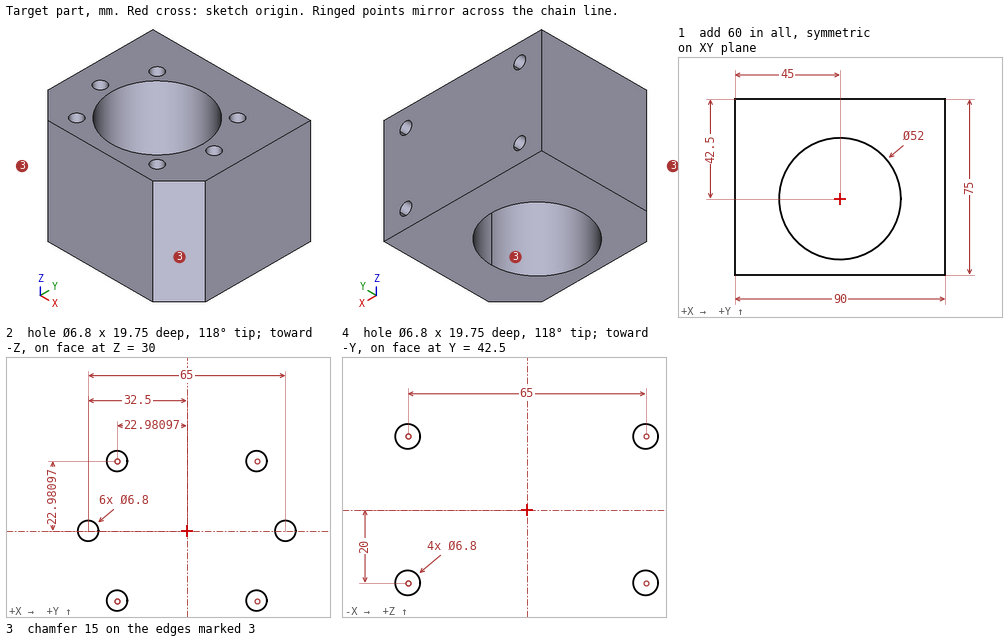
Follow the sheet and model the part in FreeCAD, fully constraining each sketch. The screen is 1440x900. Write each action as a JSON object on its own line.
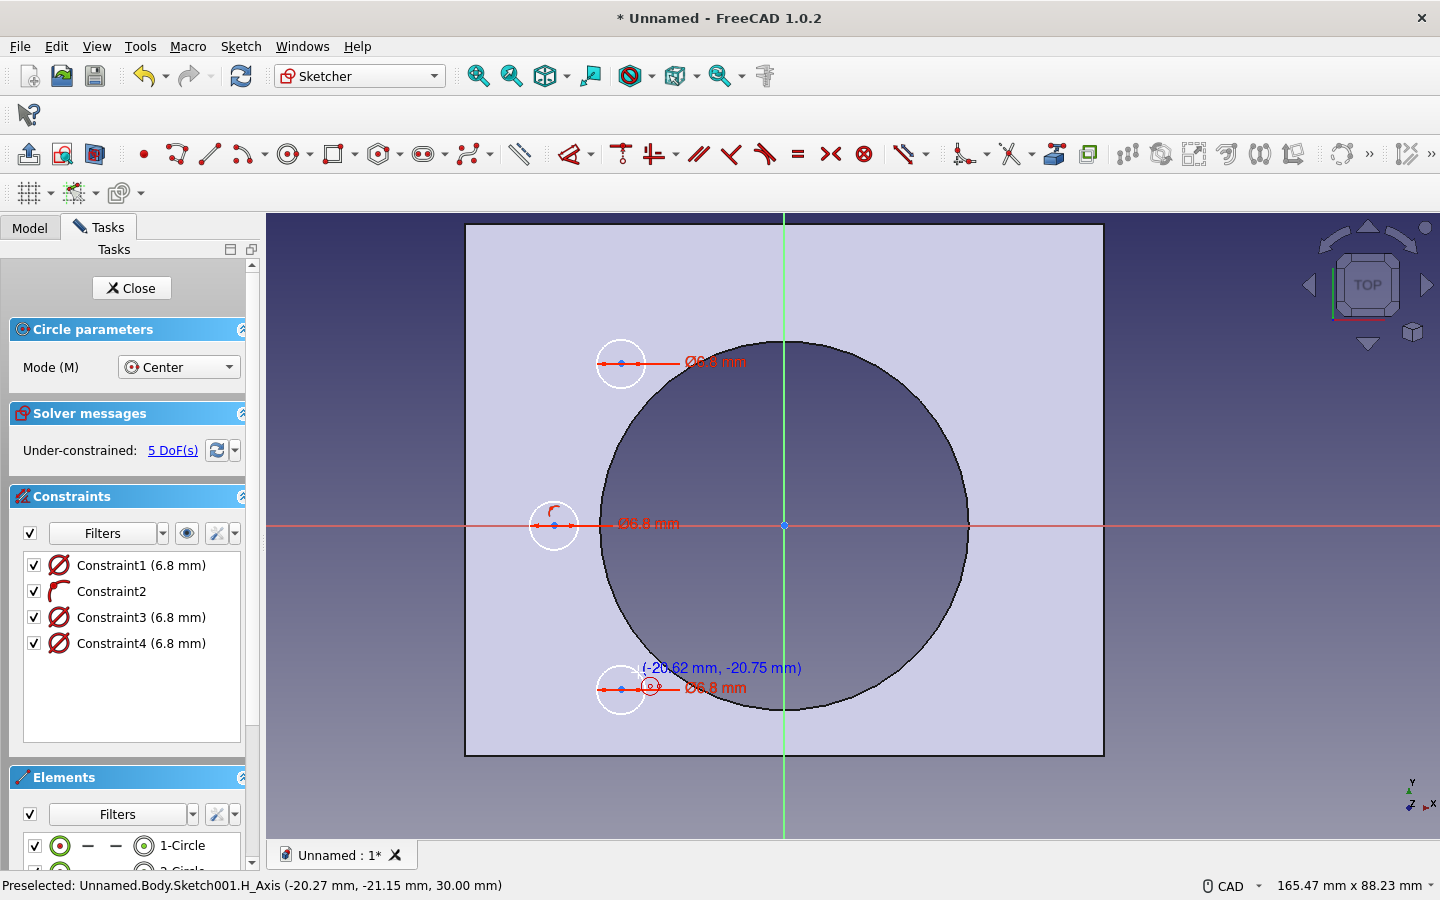
{"action": "left_click", "coordinate": [947, 689]}
{"action": "mouse_move", "coordinate": [964, 672]}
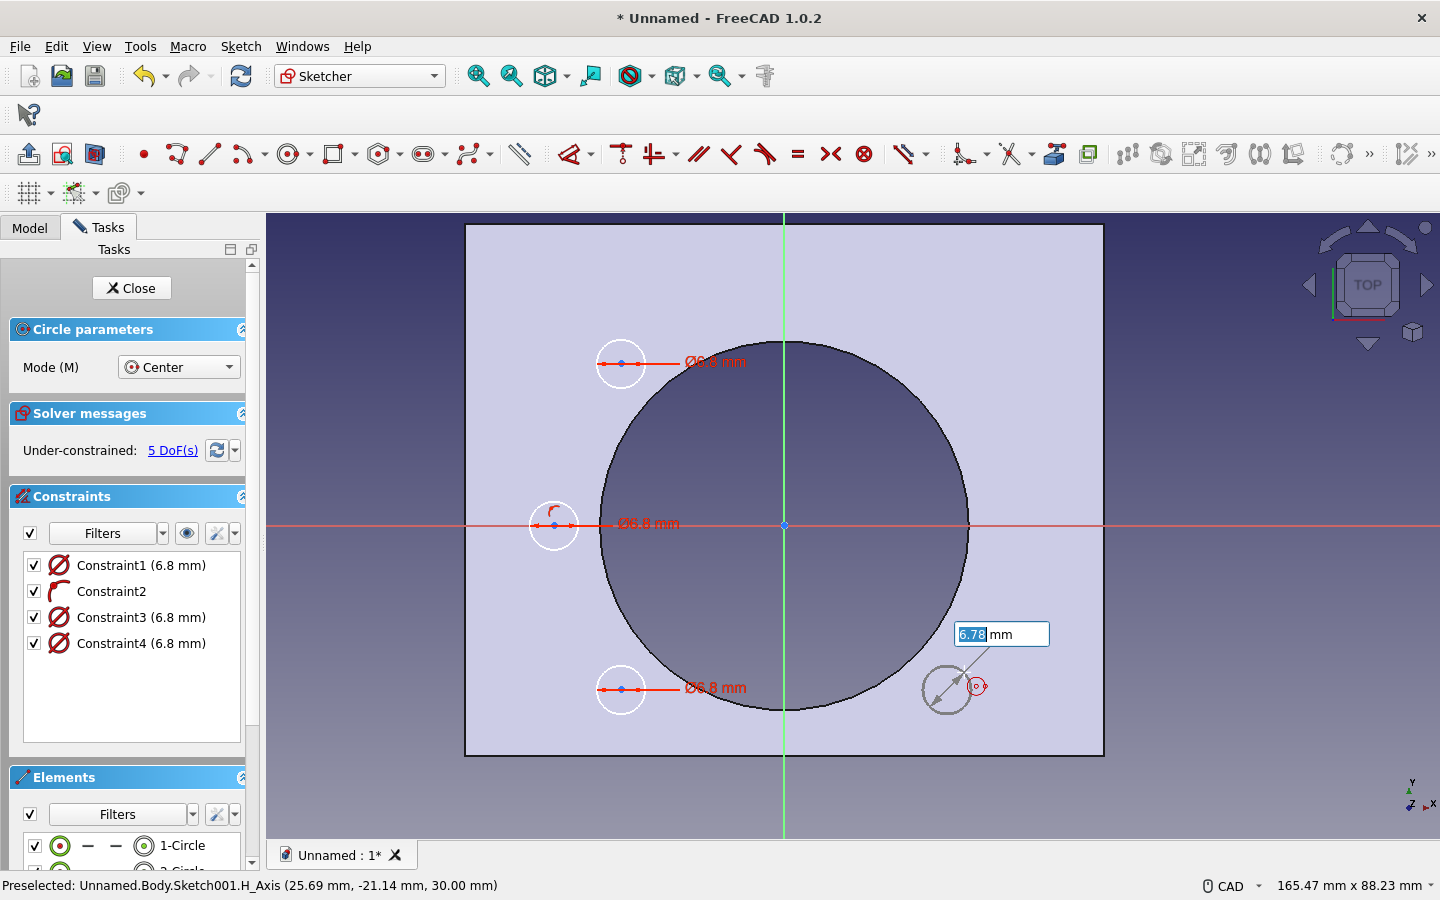
{"action": "type", "text": "6.8"}
{"action": "key", "text": "Return"}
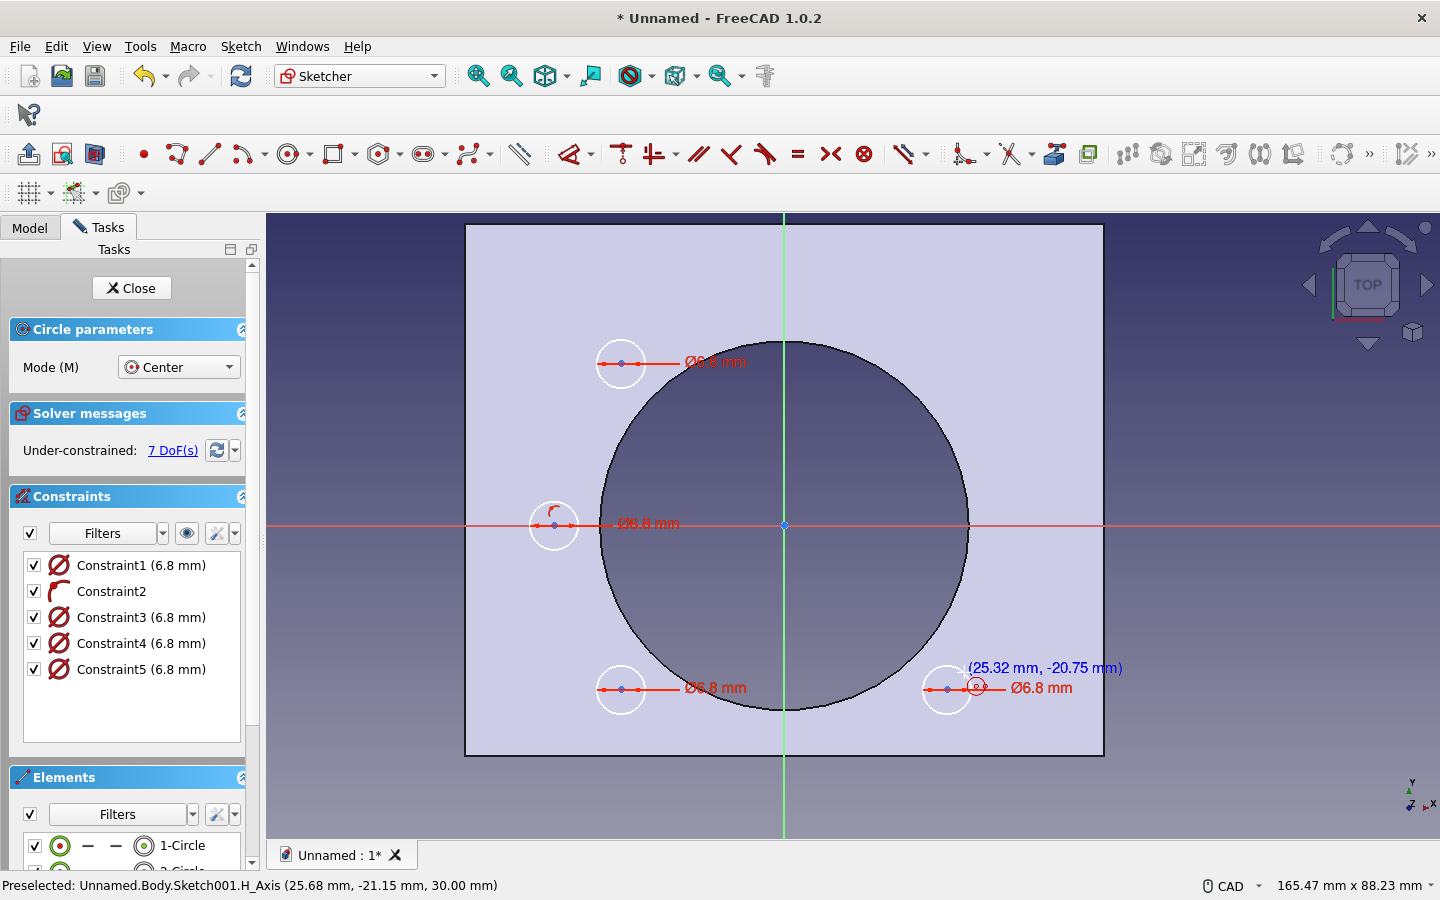
{"action": "left_click", "coordinate": [1015, 526]}
{"action": "mouse_move", "coordinate": [1032, 509]}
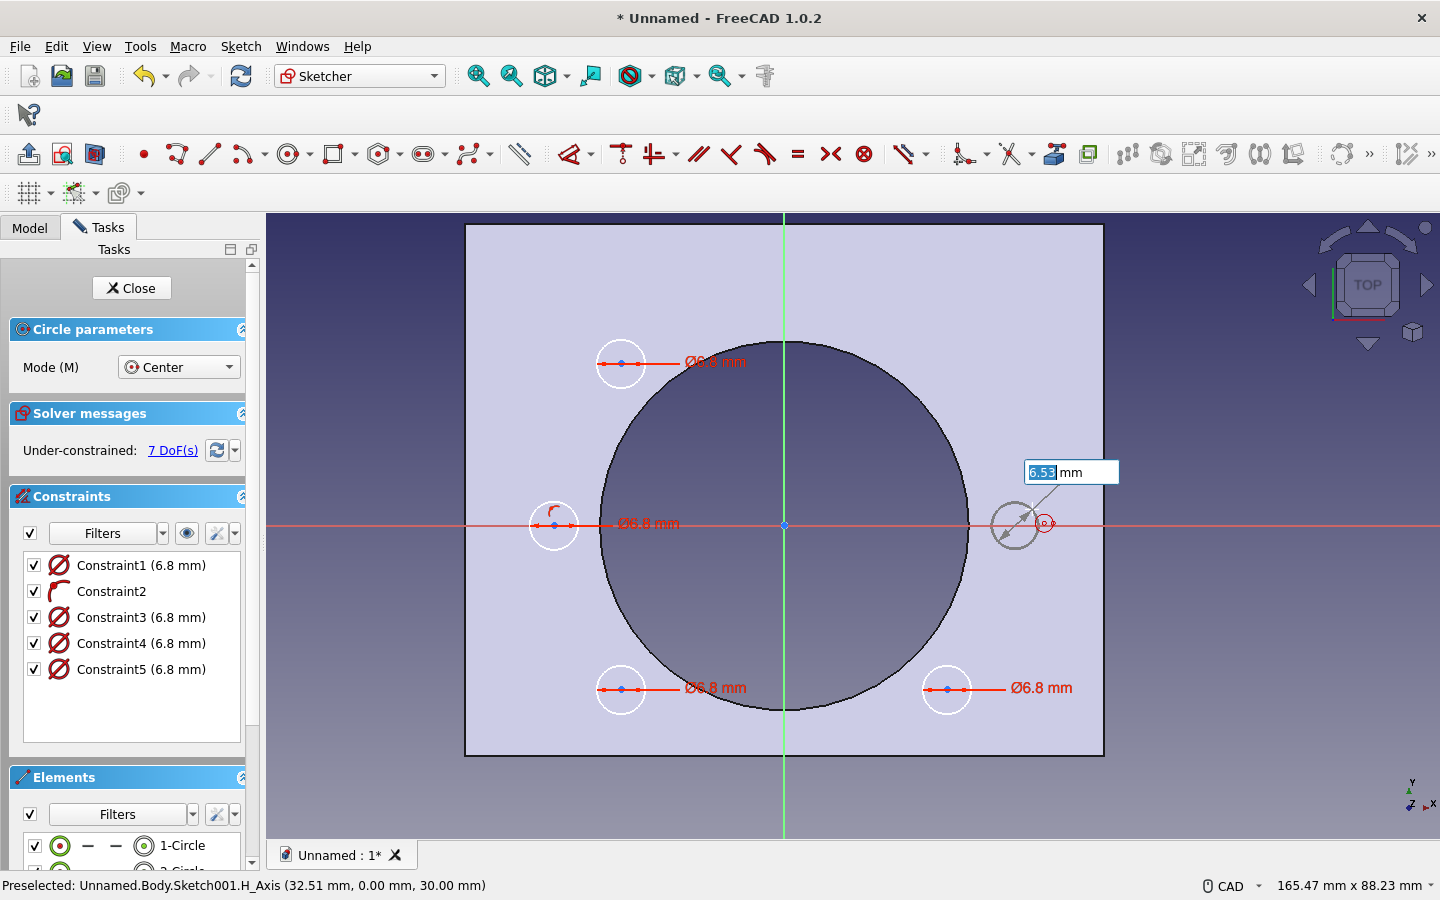
{"action": "type", "text": "6.8"}
{"action": "key", "text": "Return"}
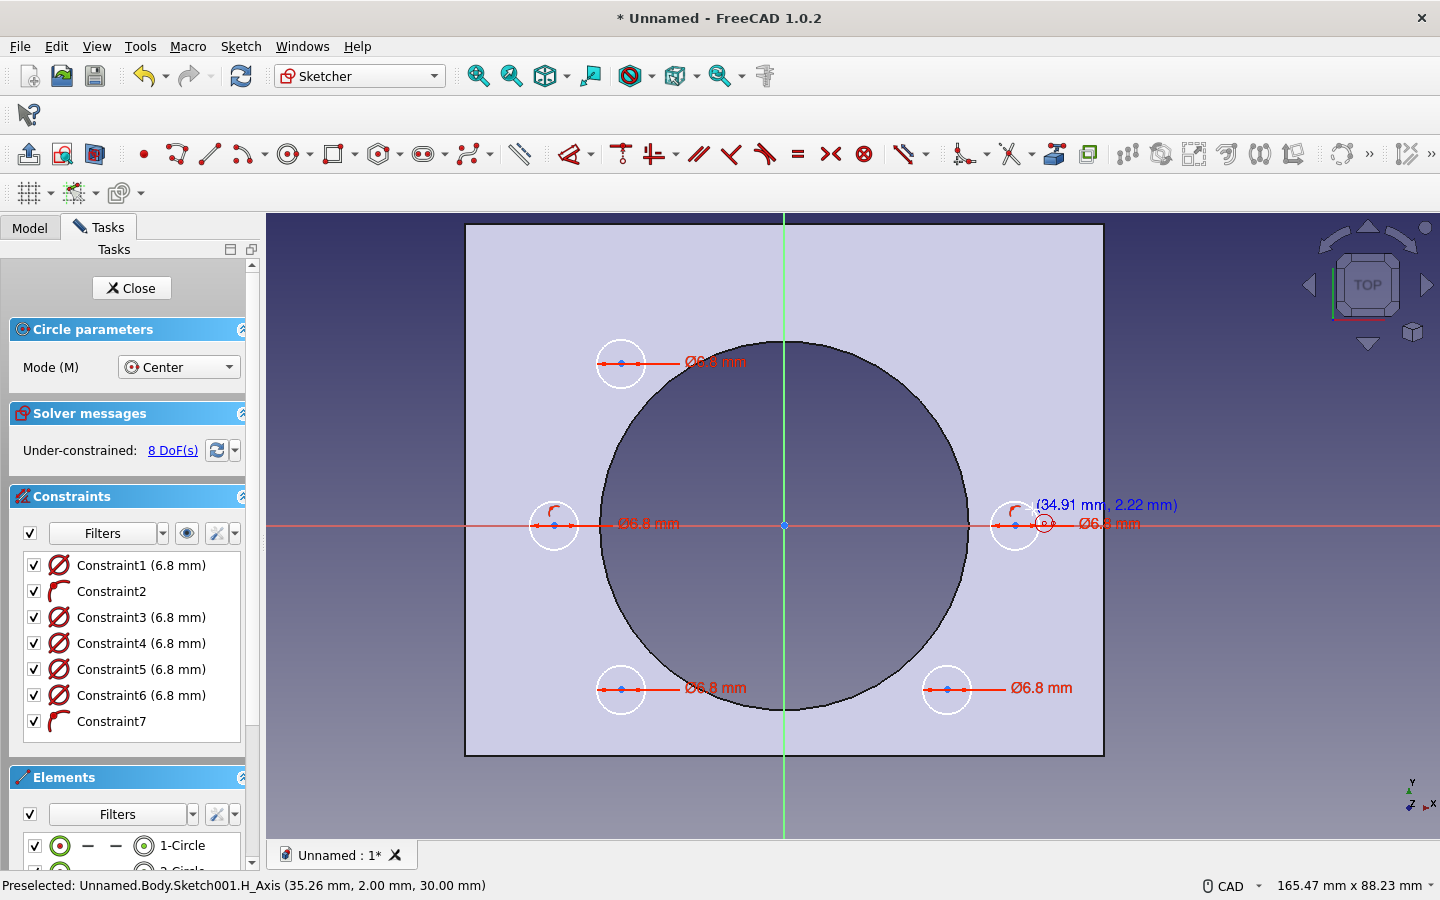
{"action": "left_click", "coordinate": [947, 363]}
{"action": "mouse_move", "coordinate": [964, 346]}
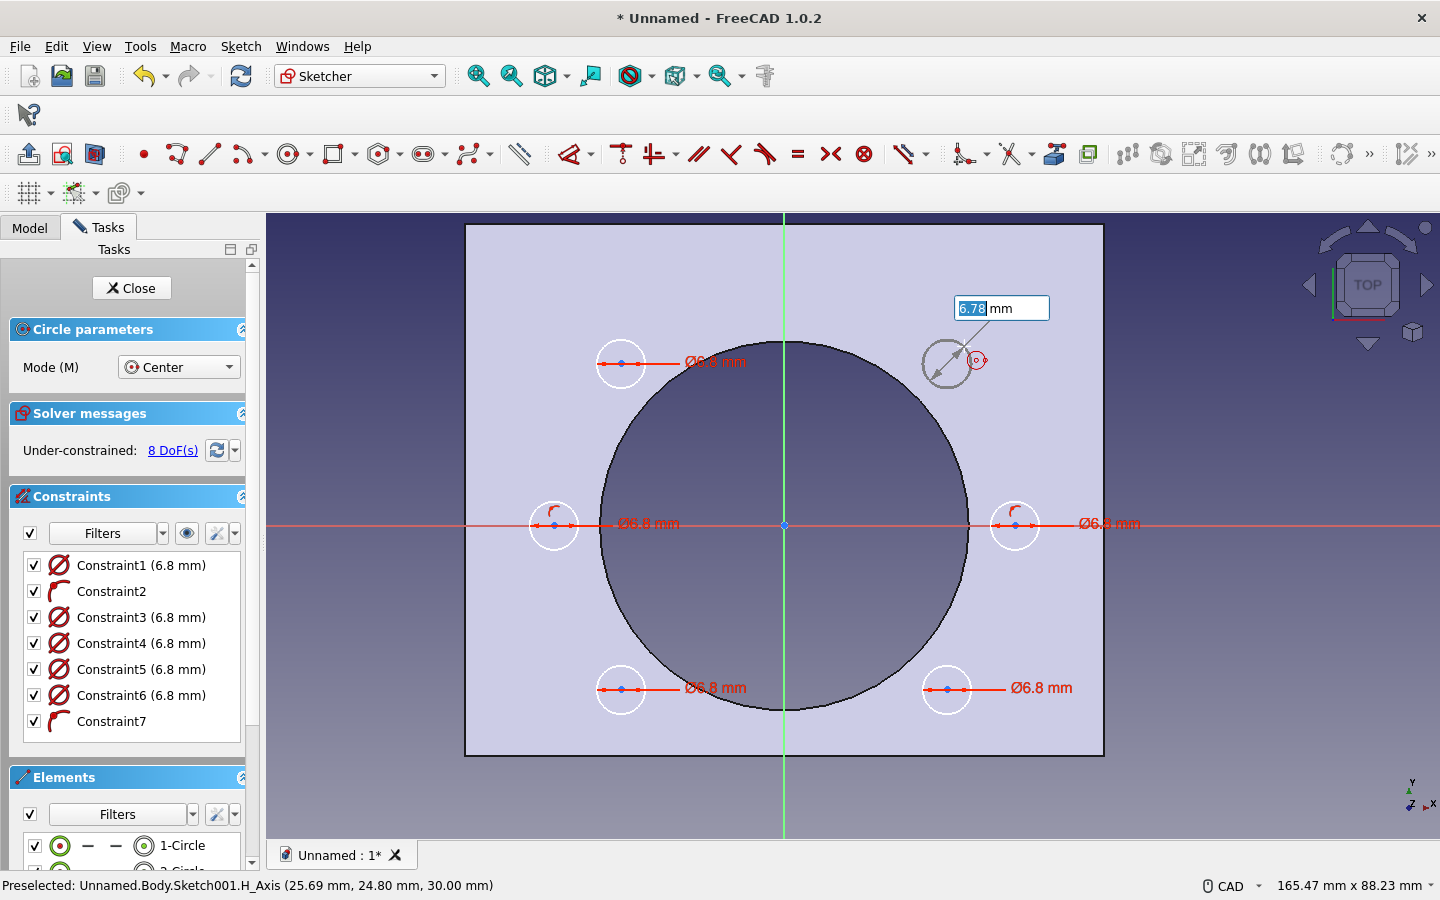
{"action": "type", "text": "6.8"}
{"action": "key", "text": "Return"}
{"action": "key", "text": "Escape"}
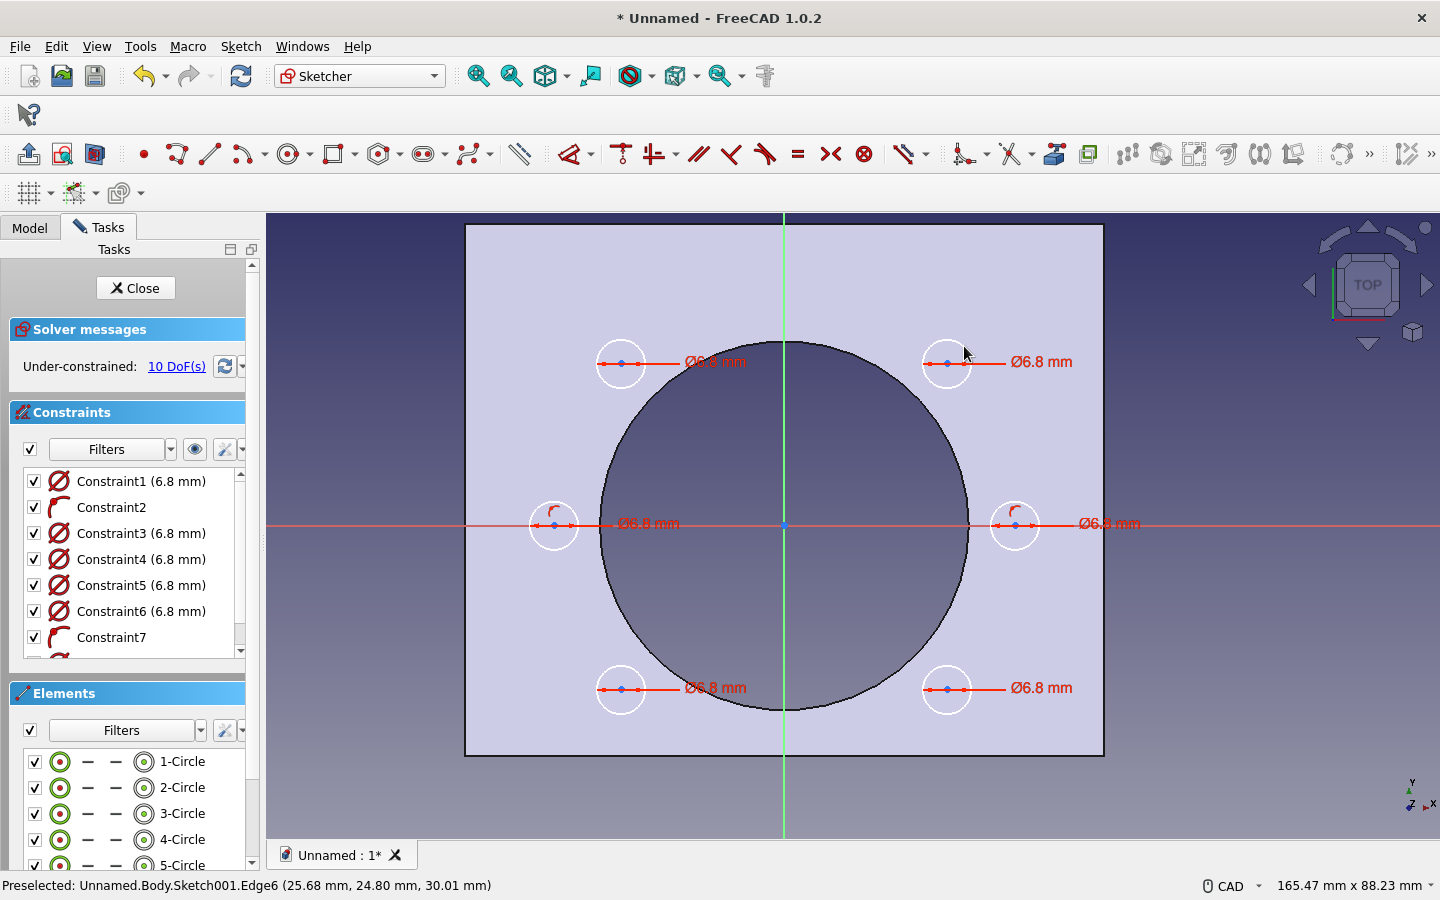
{"action": "left_click", "coordinate": [621, 364]}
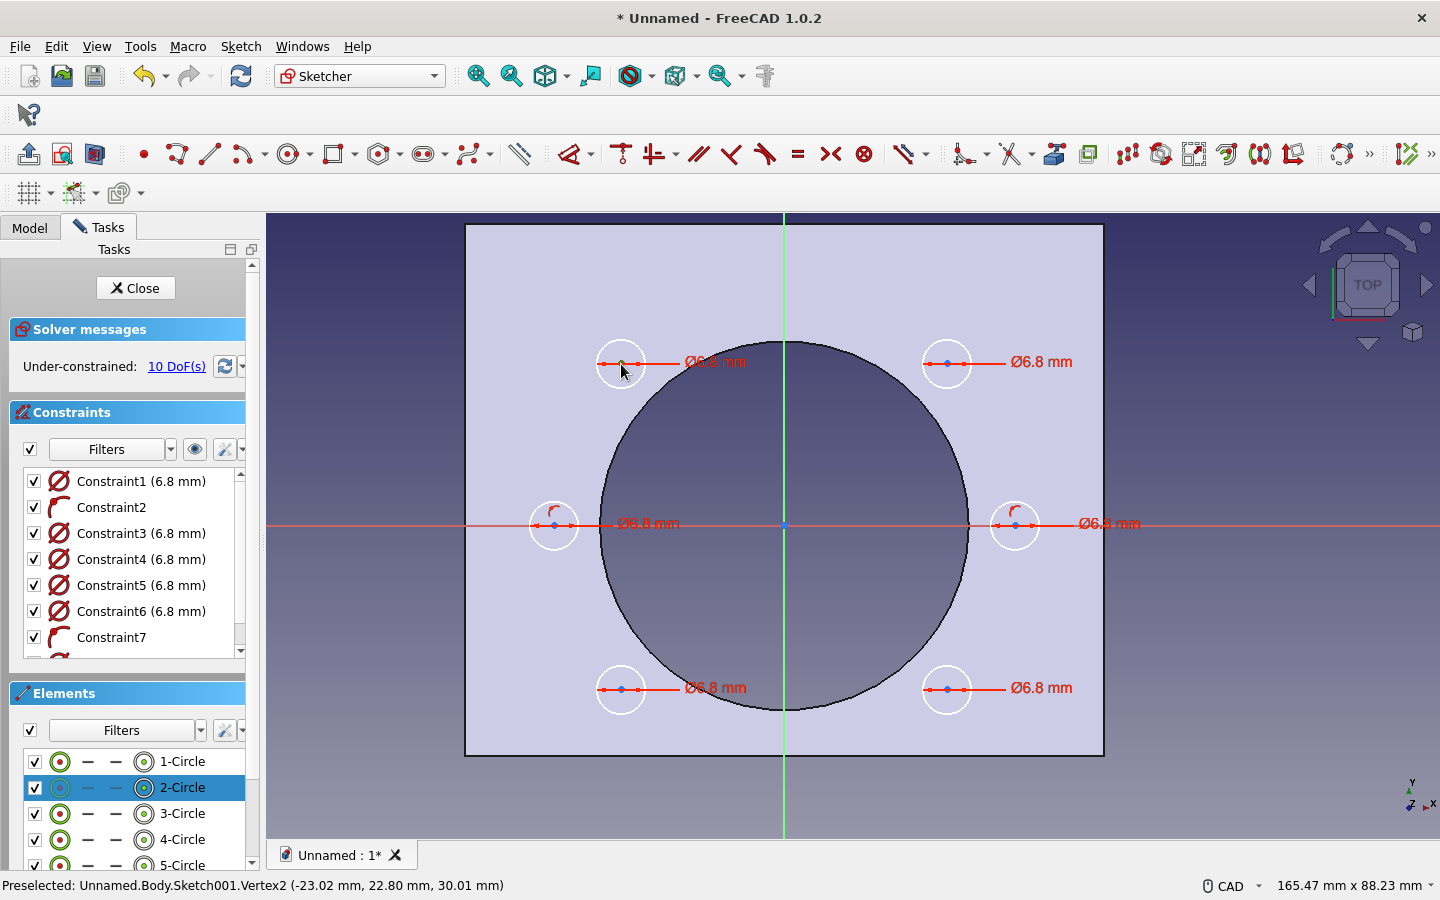
{"action": "left_click", "coordinate": [621, 690]}